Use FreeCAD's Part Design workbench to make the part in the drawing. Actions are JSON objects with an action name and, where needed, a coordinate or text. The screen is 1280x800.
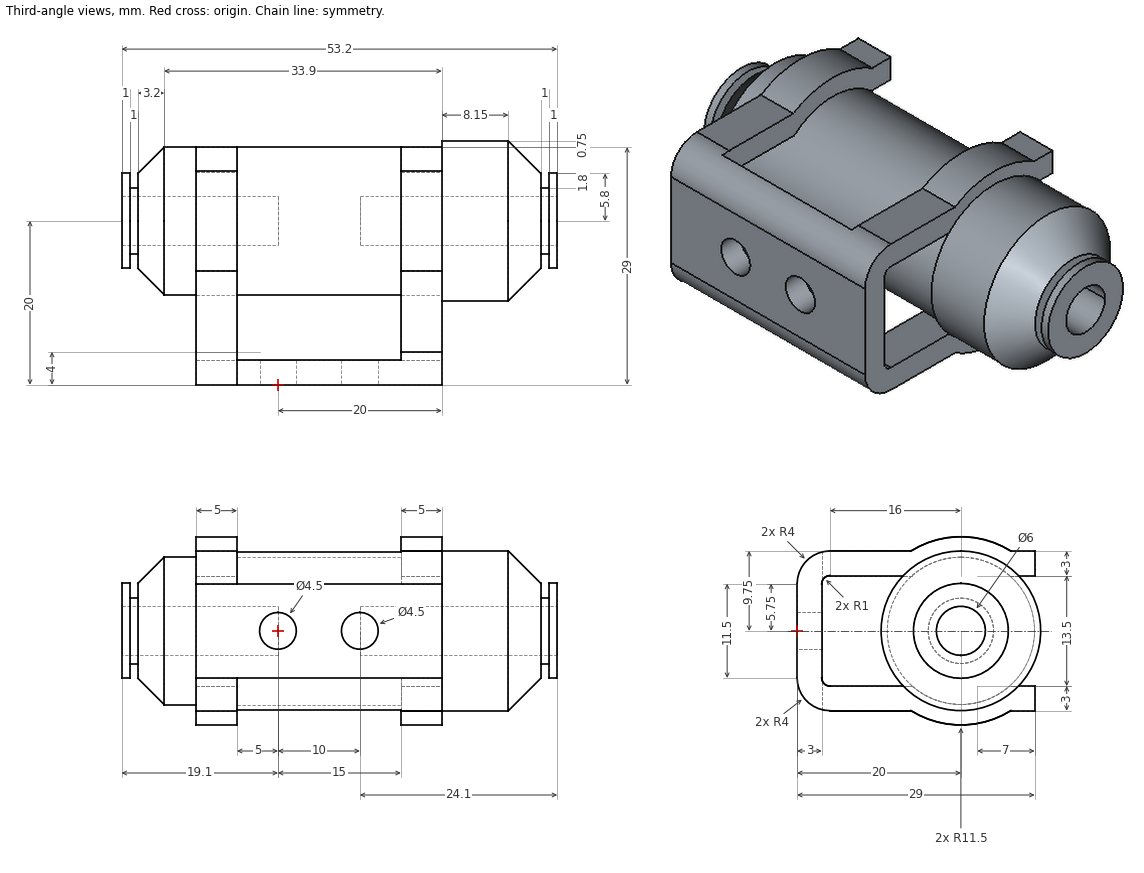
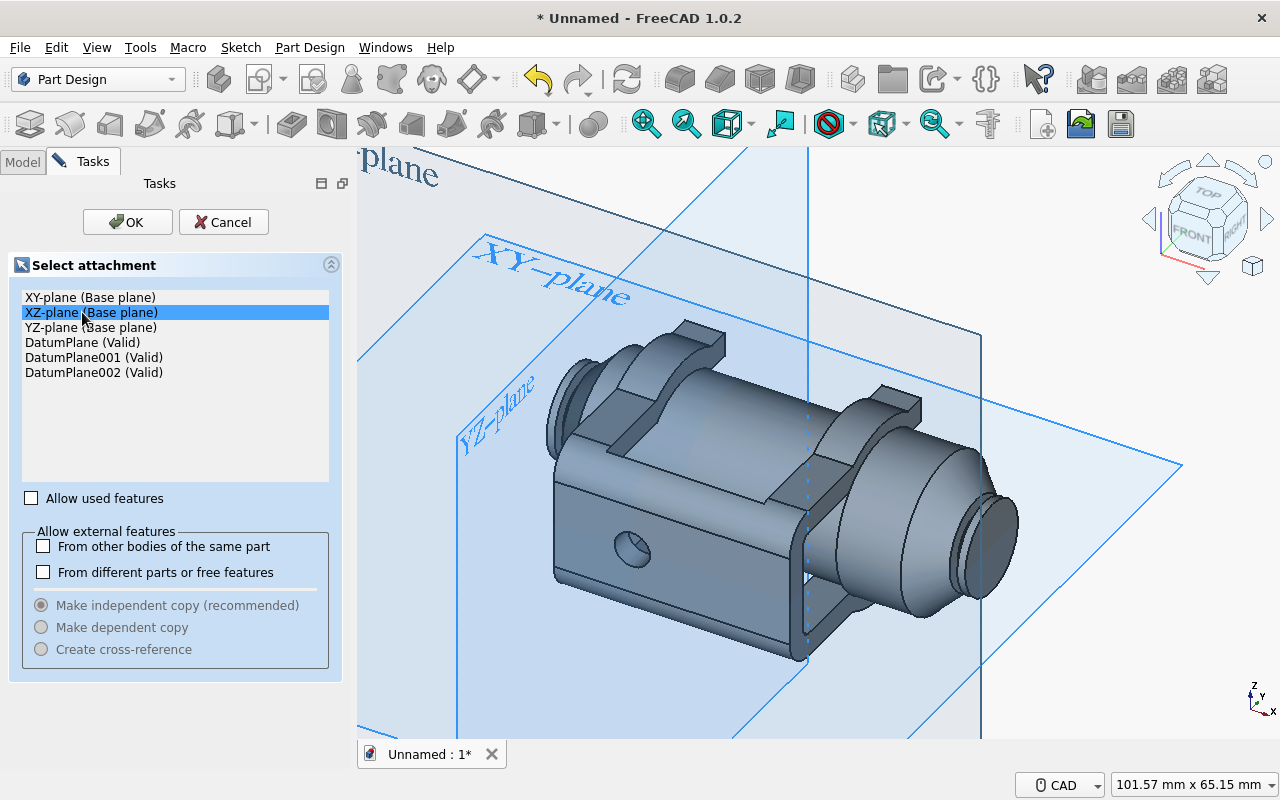
{"action": "left_click", "coordinate": [128, 222]}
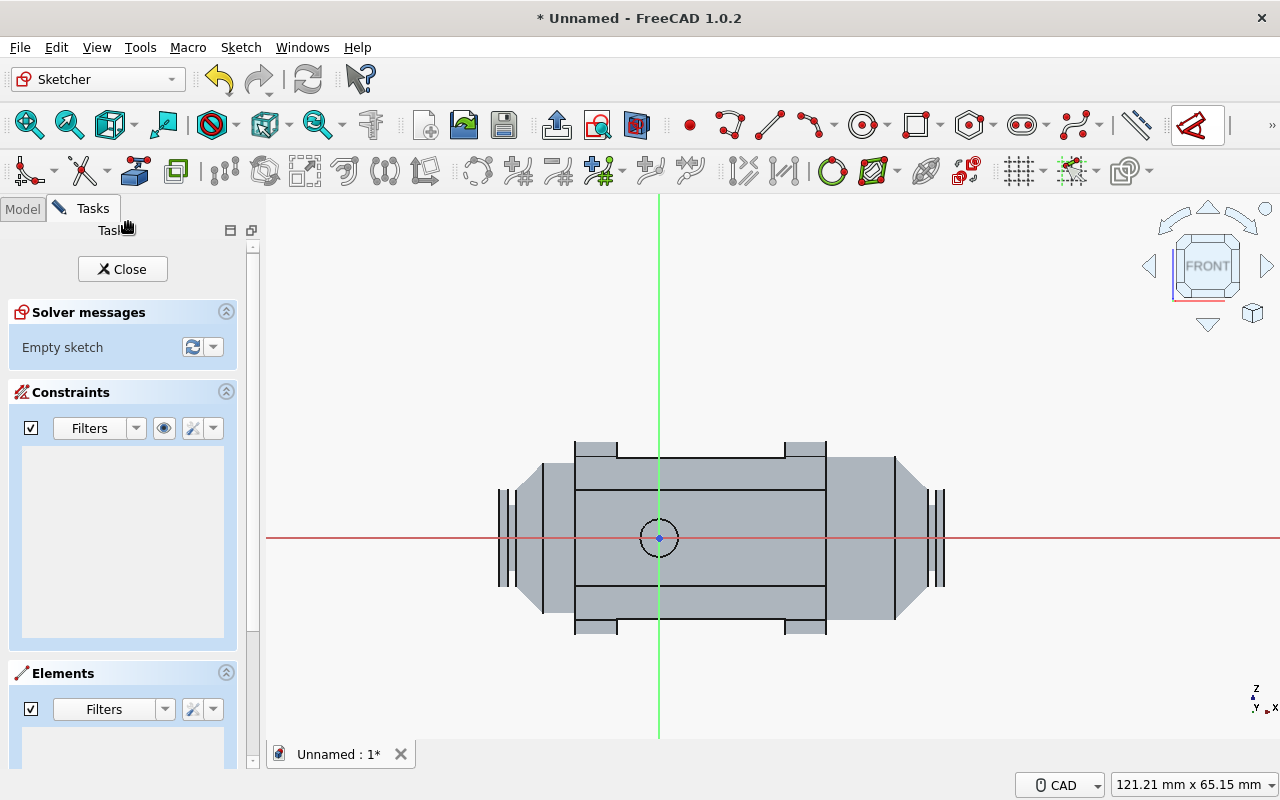
{"action": "scroll", "coordinate": [748, 547], "scroll_direction": "up", "scroll_amount": 11}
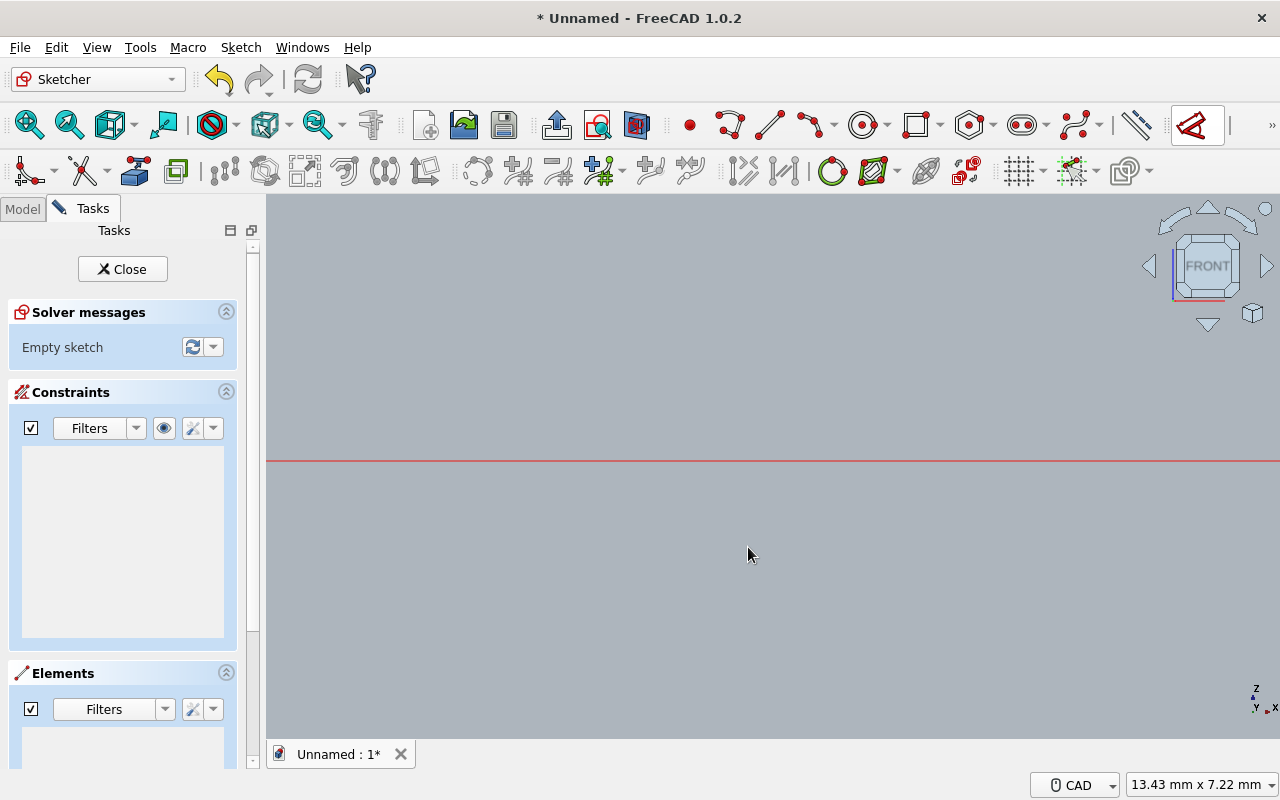
{"action": "left_click", "coordinate": [864, 126]}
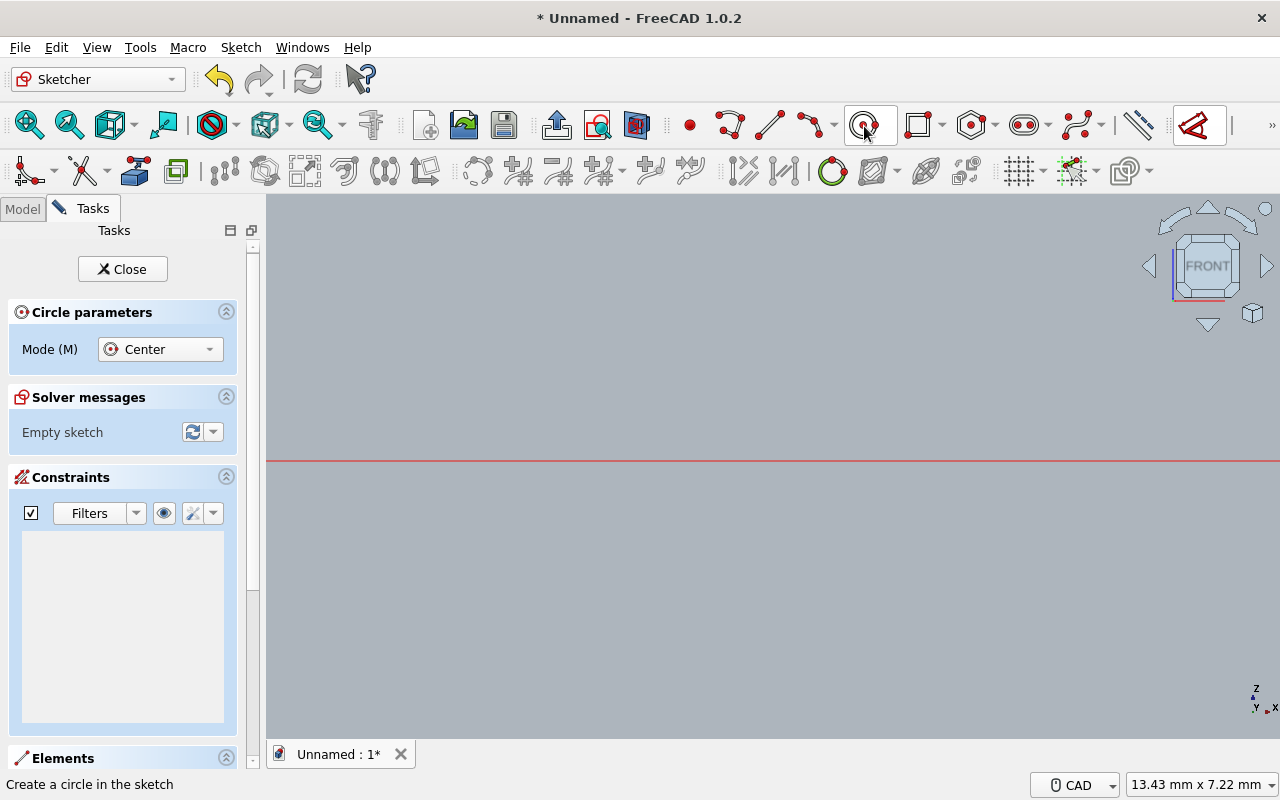
{"action": "left_click", "coordinate": [697, 461]}
{"action": "left_click", "coordinate": [817, 341]}
{"action": "key", "text": "Escape"}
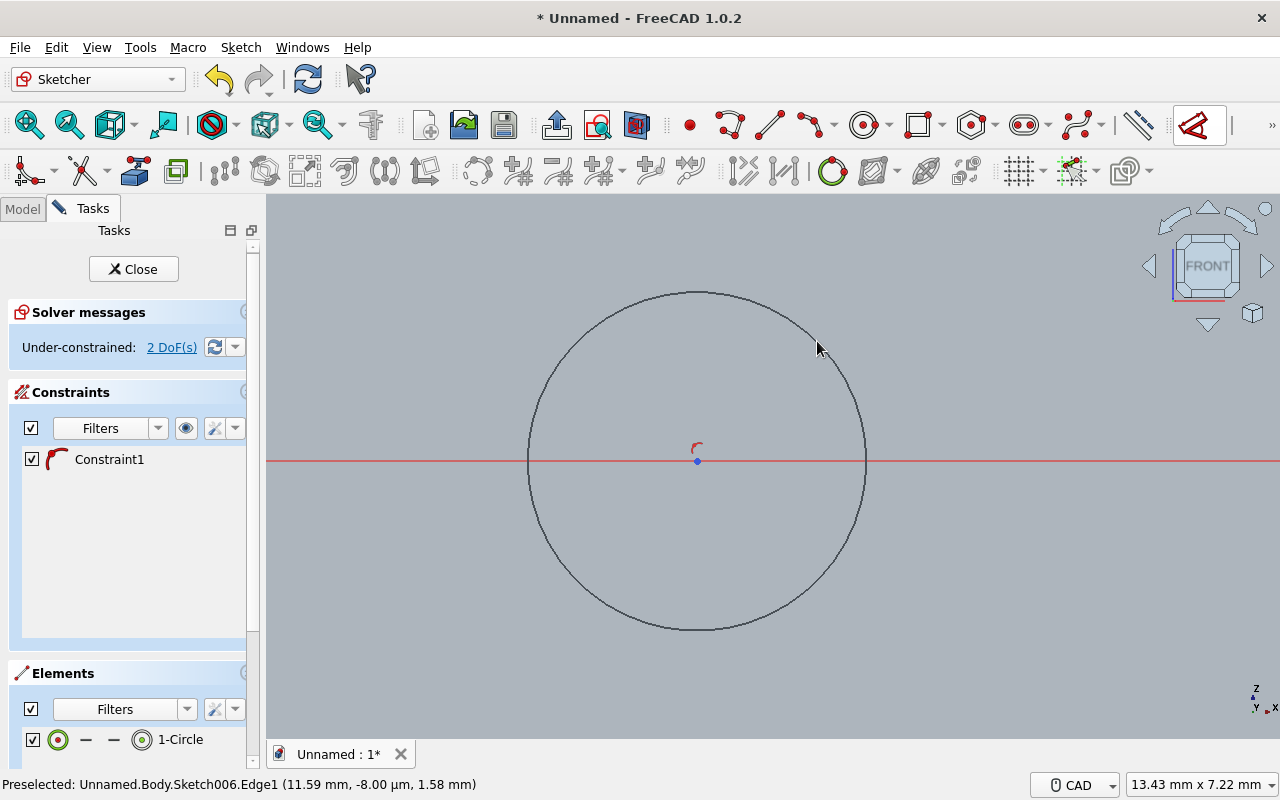
{"action": "left_click", "coordinate": [816, 341]}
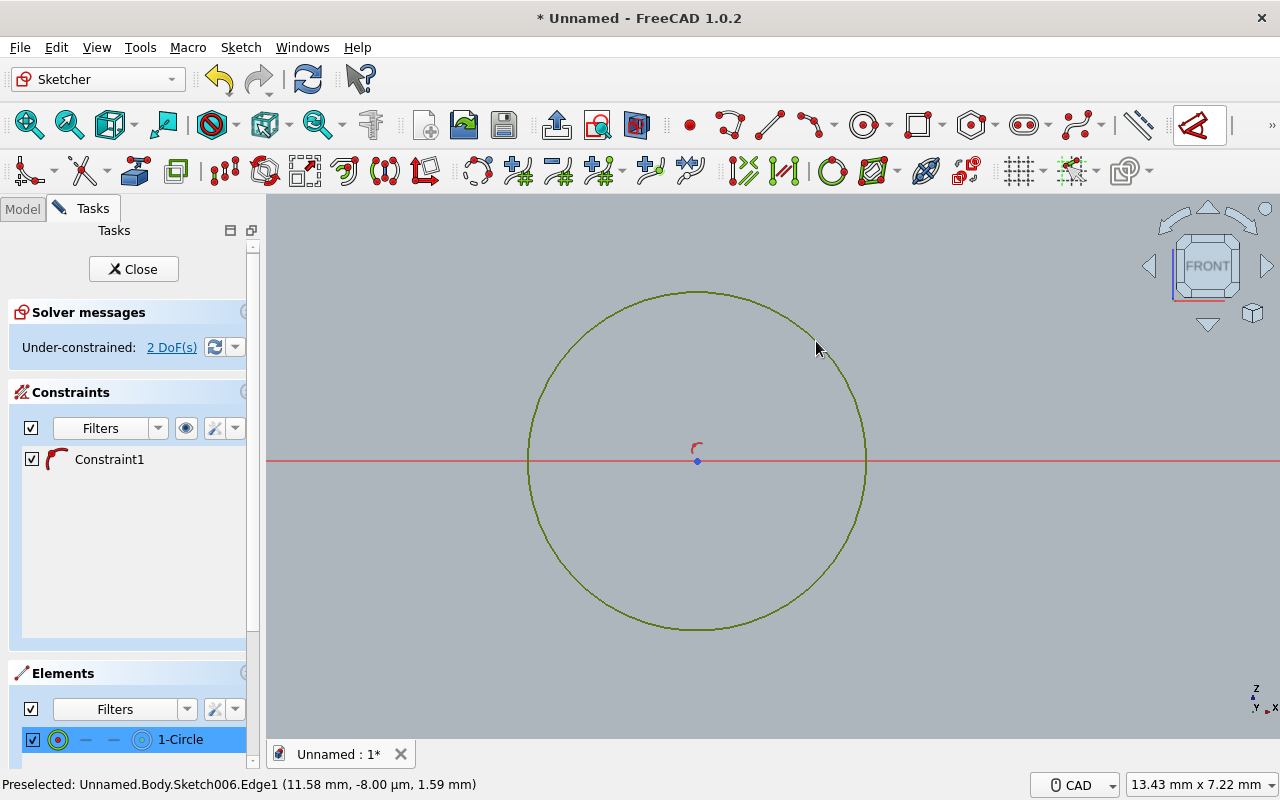
{"action": "left_click", "coordinate": [1220, 126]}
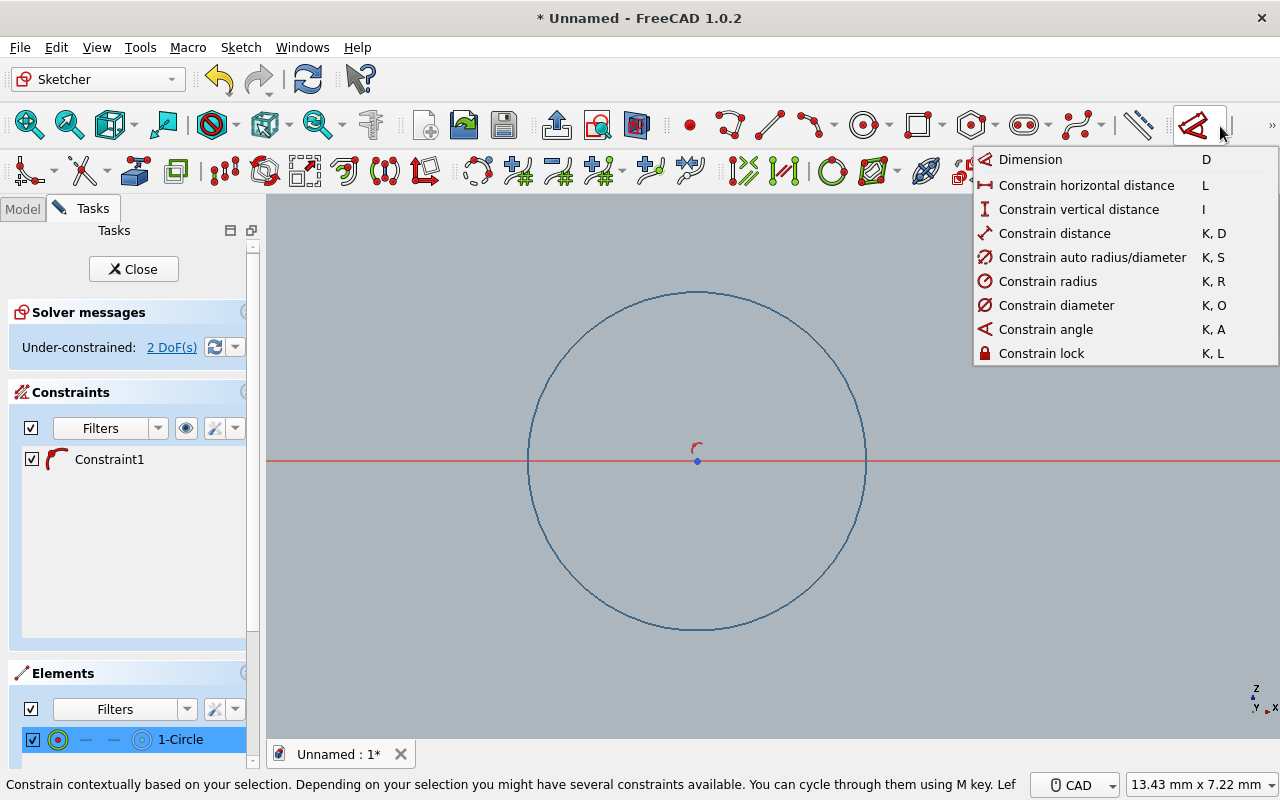
{"action": "left_click", "coordinate": [1126, 305]}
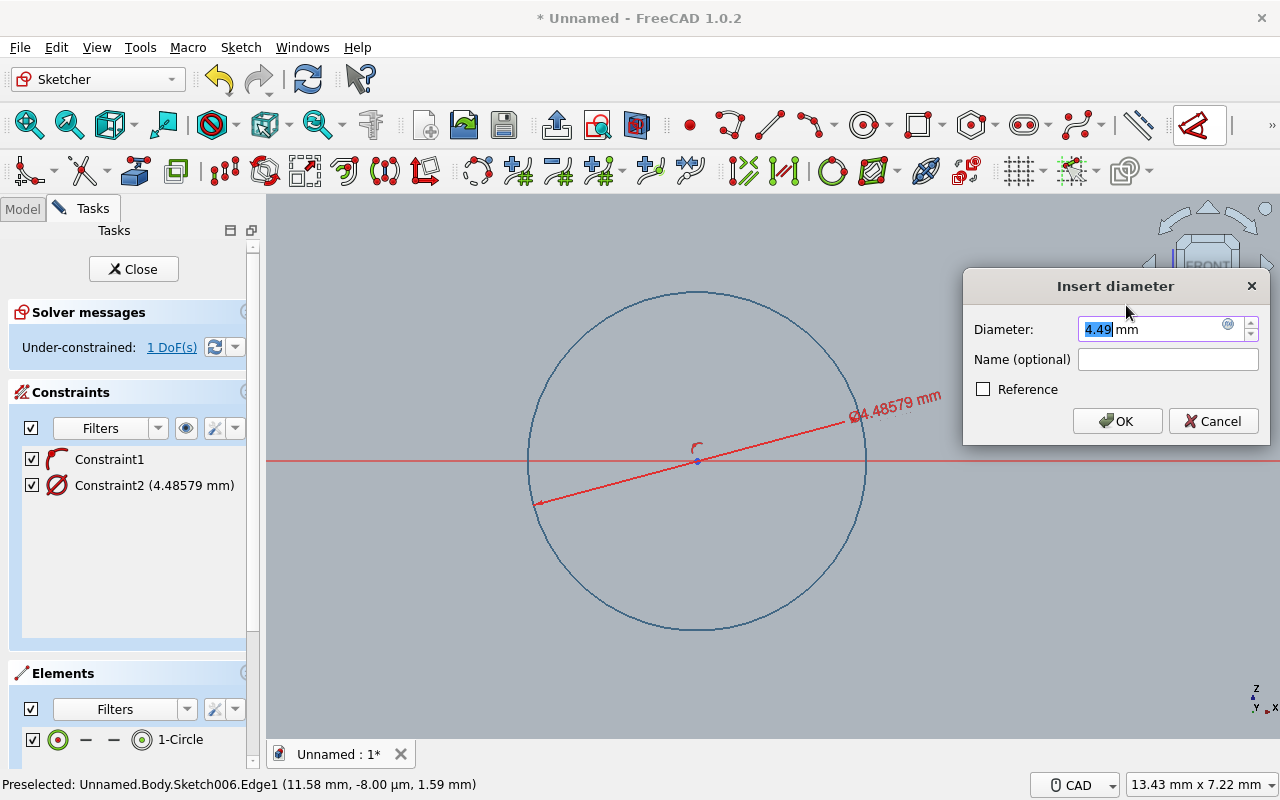
{"action": "type", "text": "4.5"}
{"action": "key", "text": "Return"}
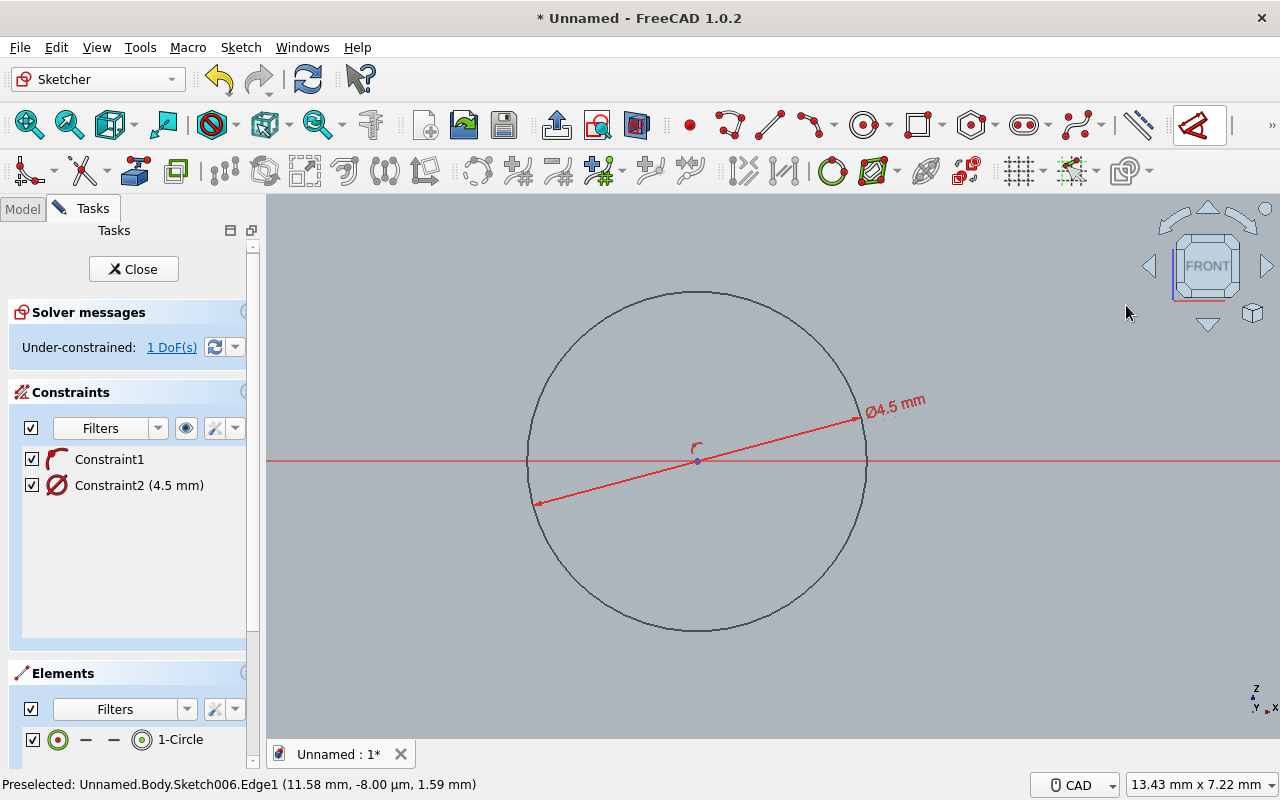
{"action": "left_click", "coordinate": [697, 461]}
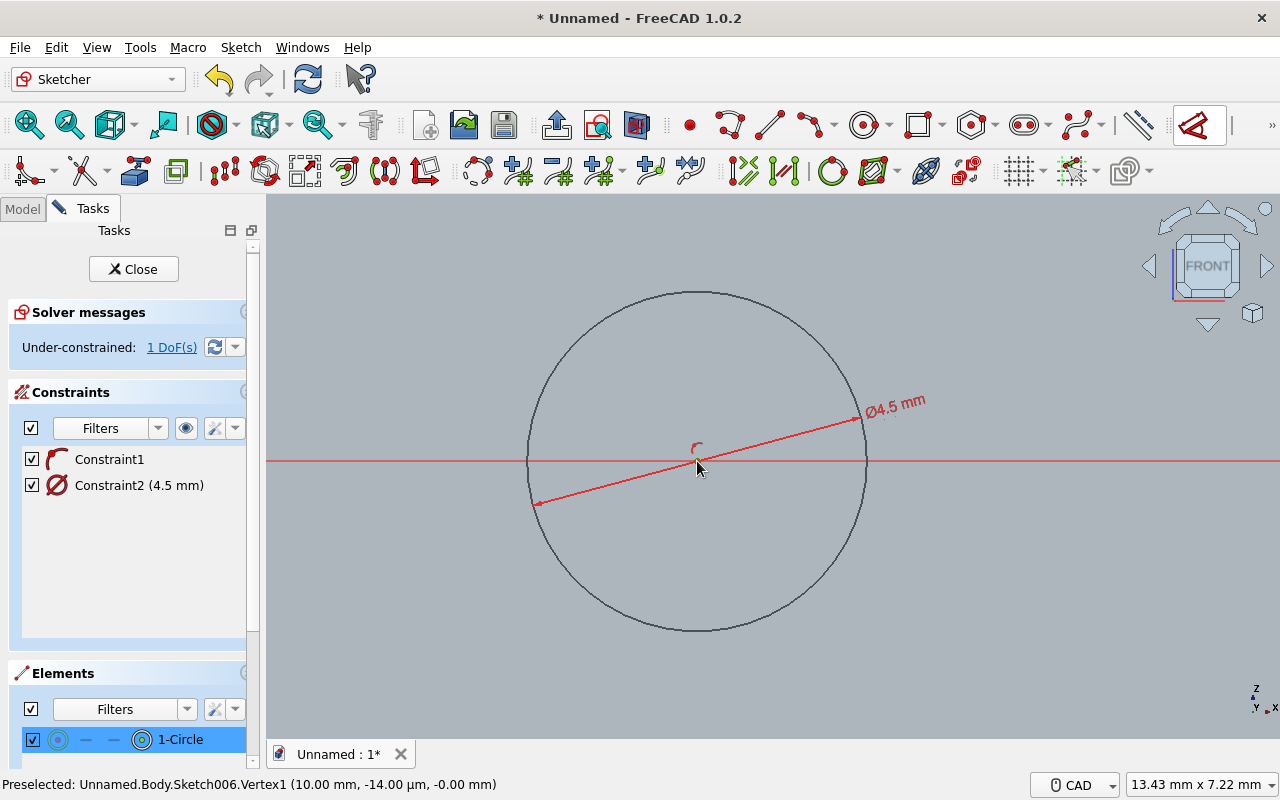
{"action": "key", "text": "l"}